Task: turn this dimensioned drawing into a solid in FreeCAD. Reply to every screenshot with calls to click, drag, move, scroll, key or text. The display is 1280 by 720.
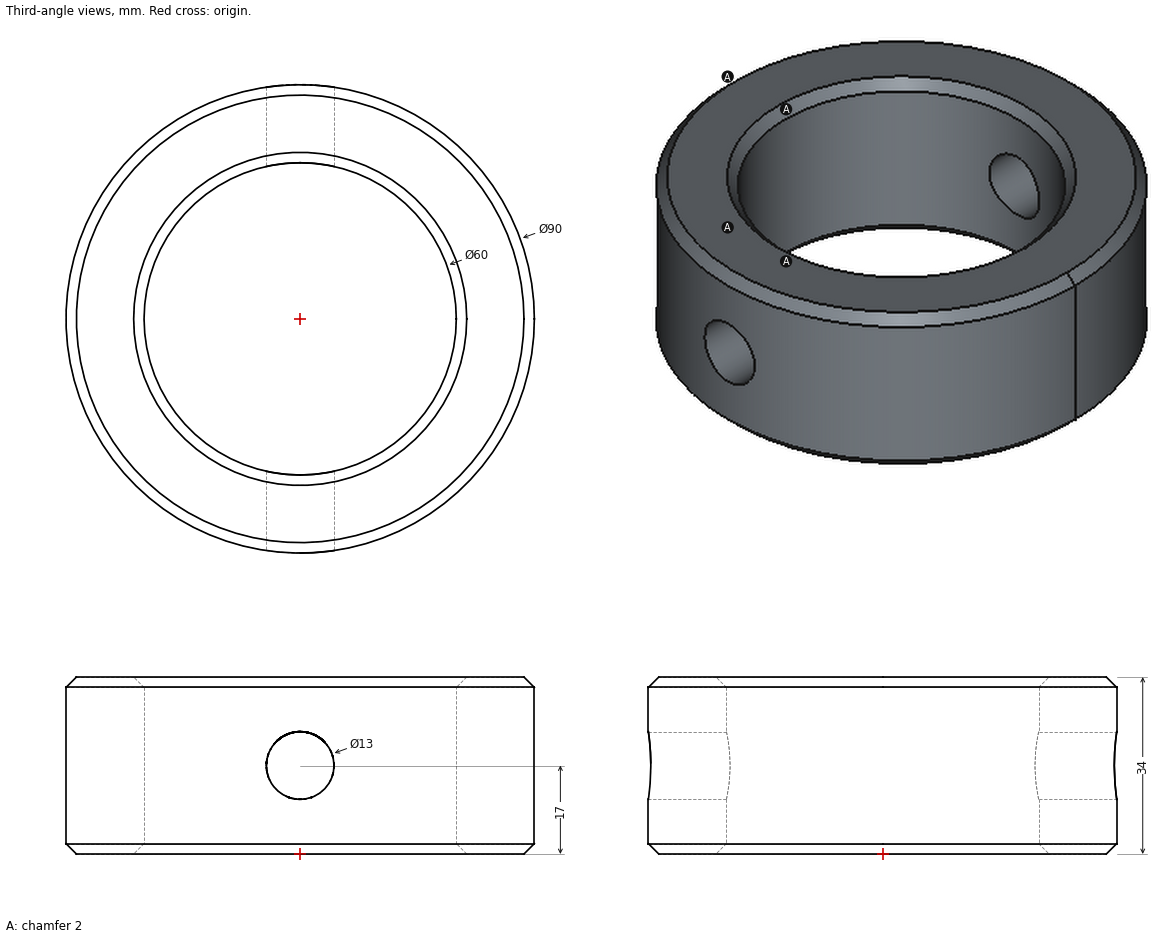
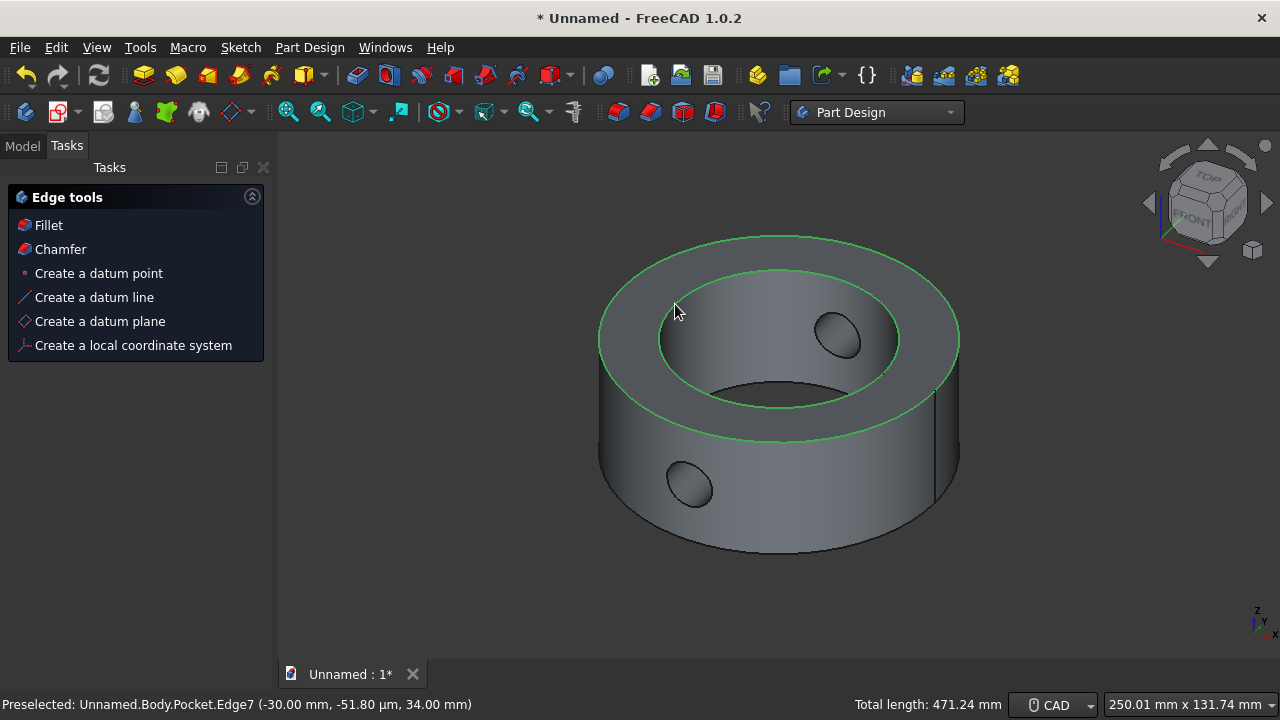
key(0)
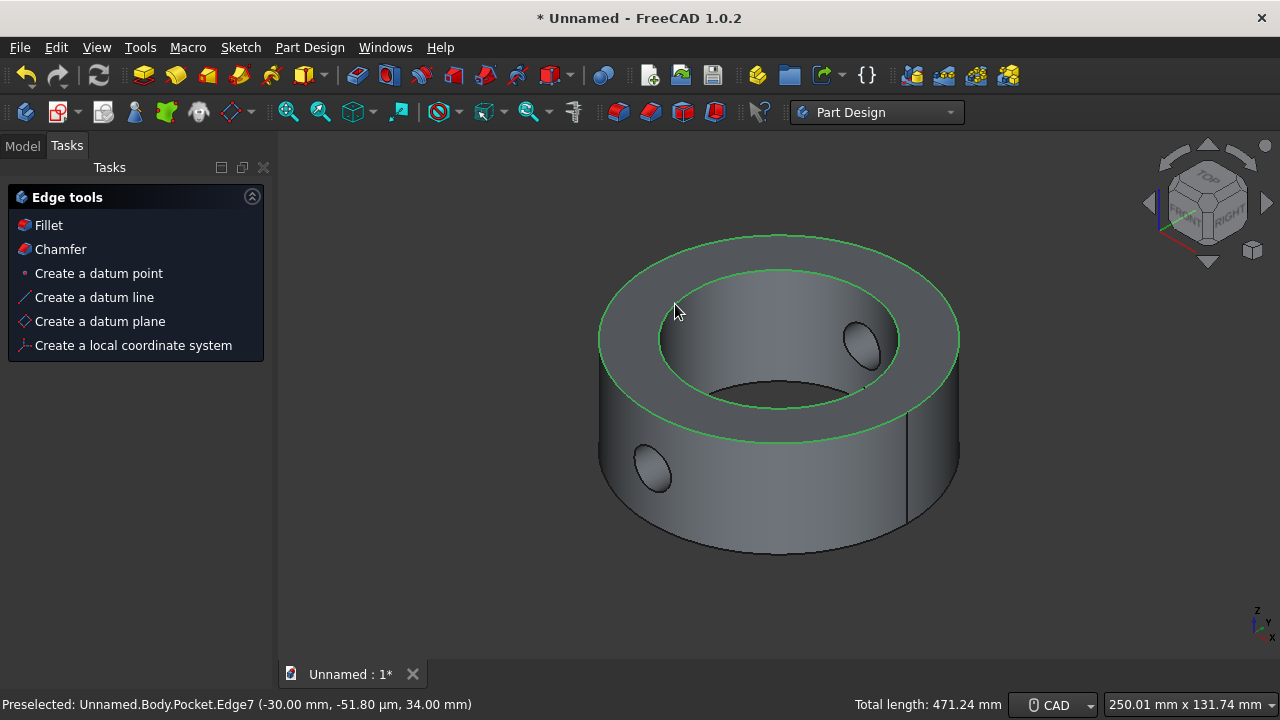
key(2)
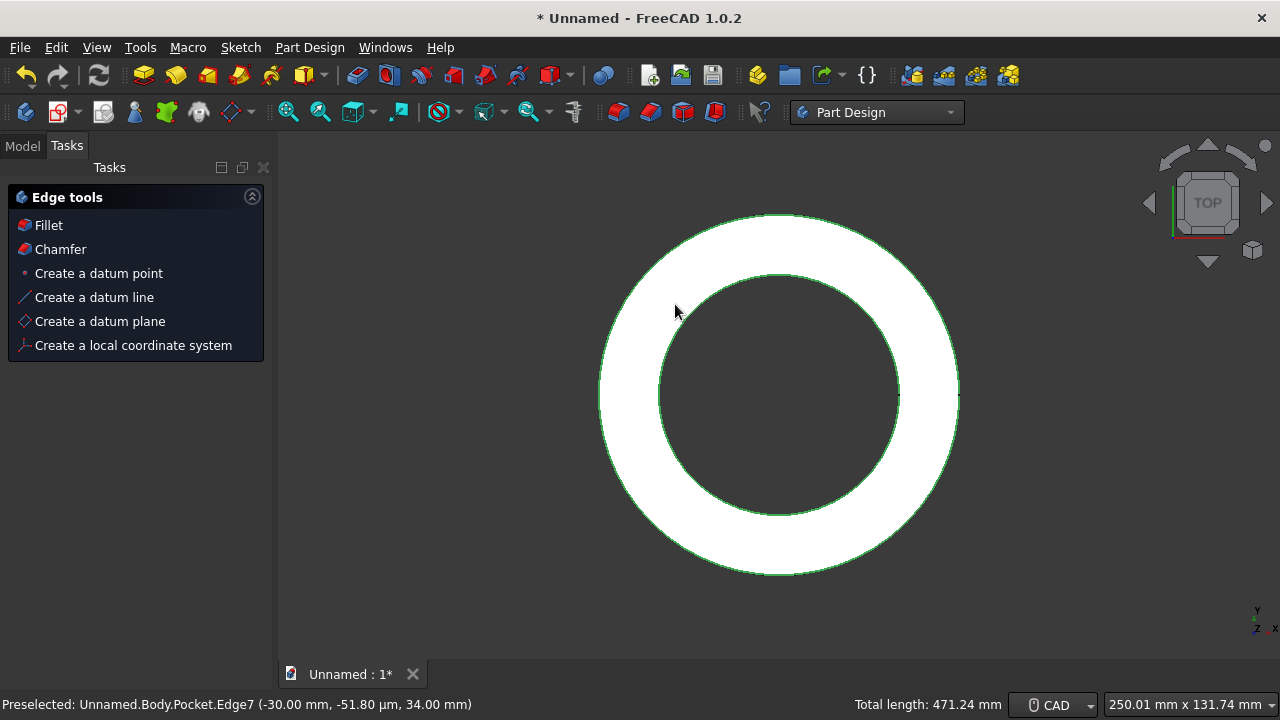
key(1)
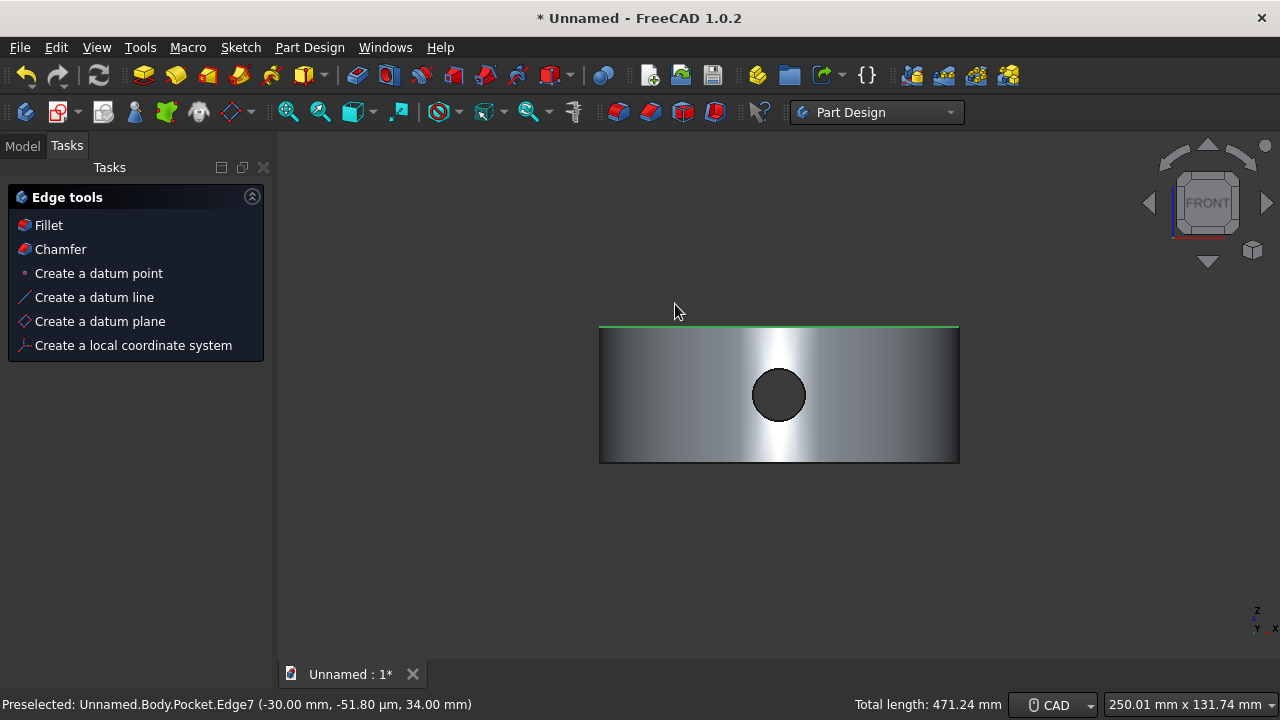
click(290, 112)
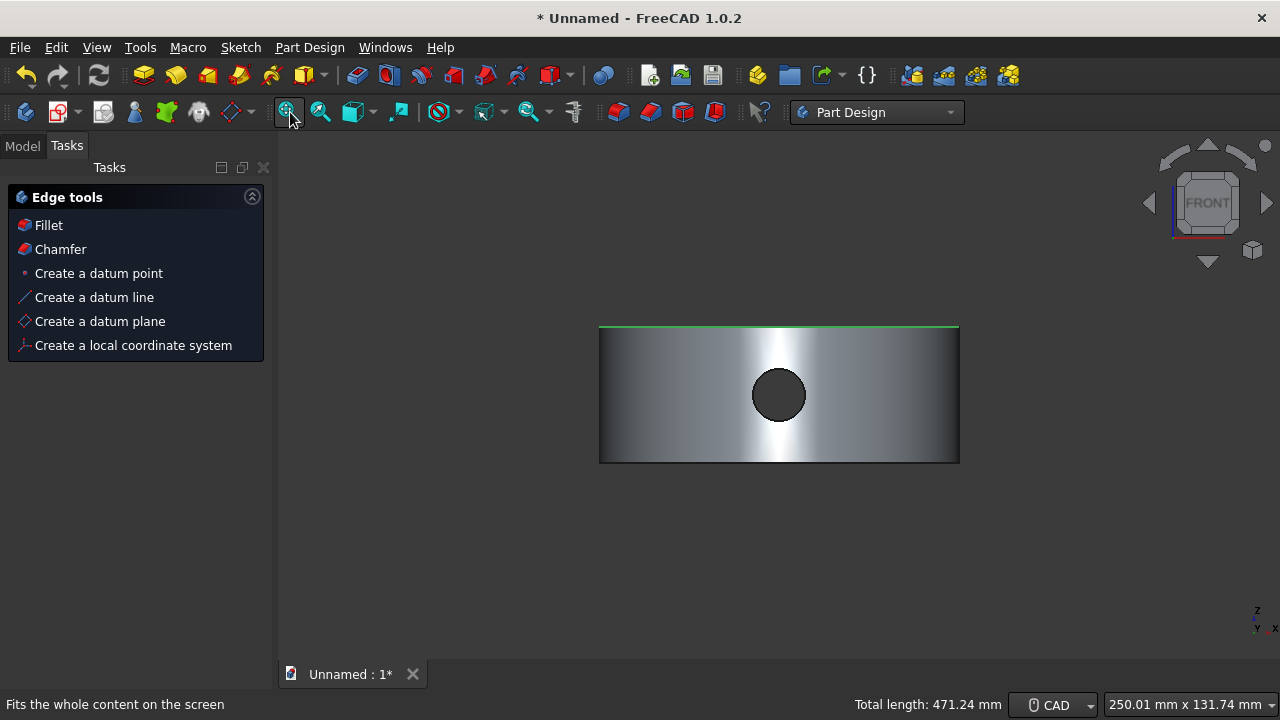
click(633, 462, ctrl)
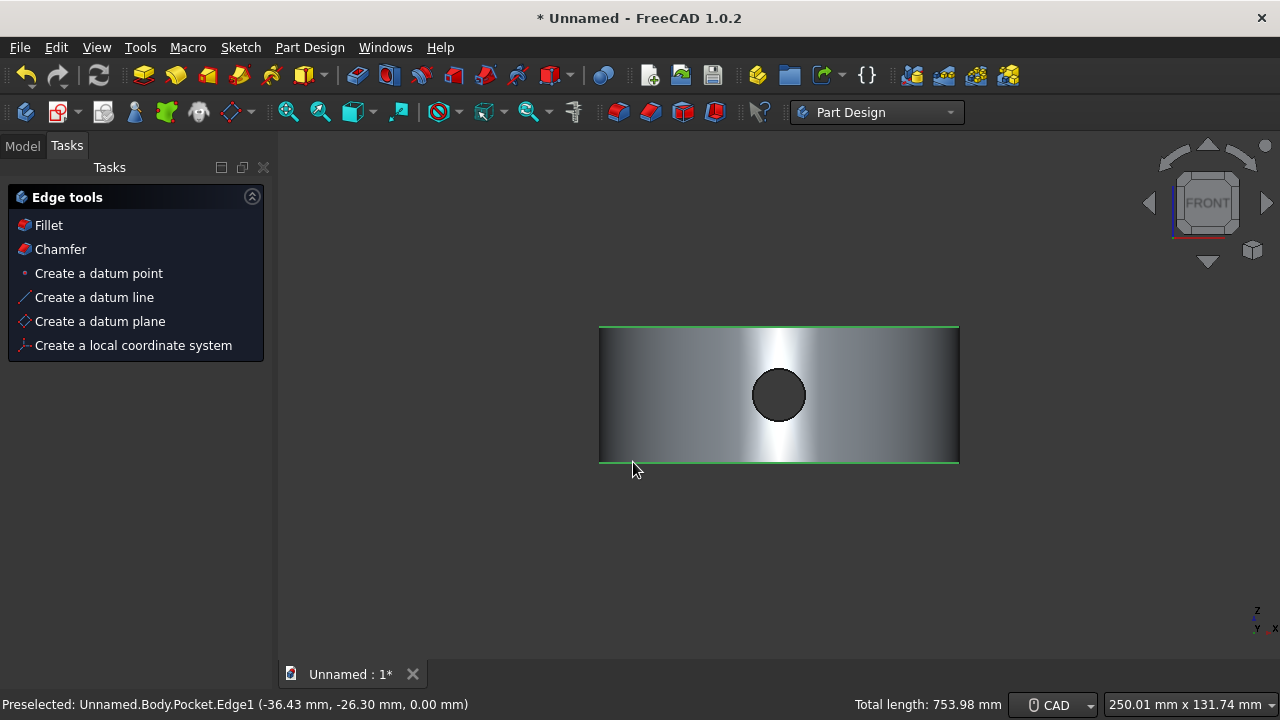
key(3)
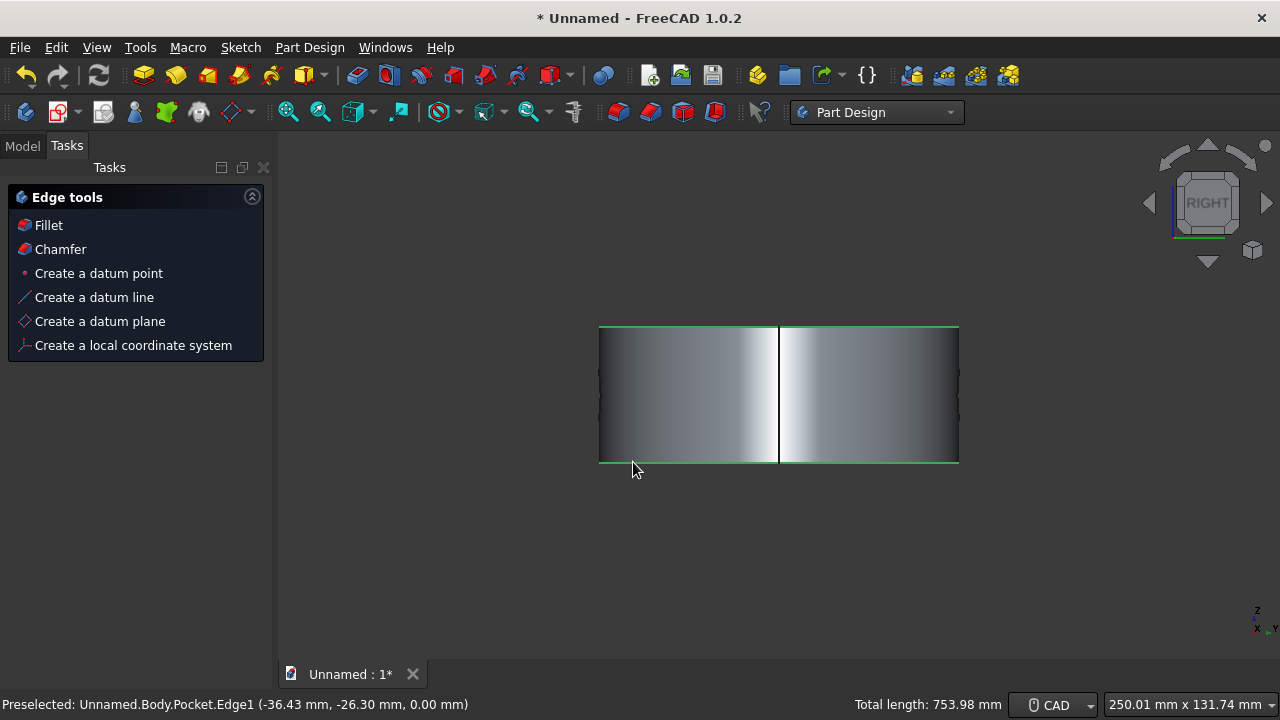
click(290, 112)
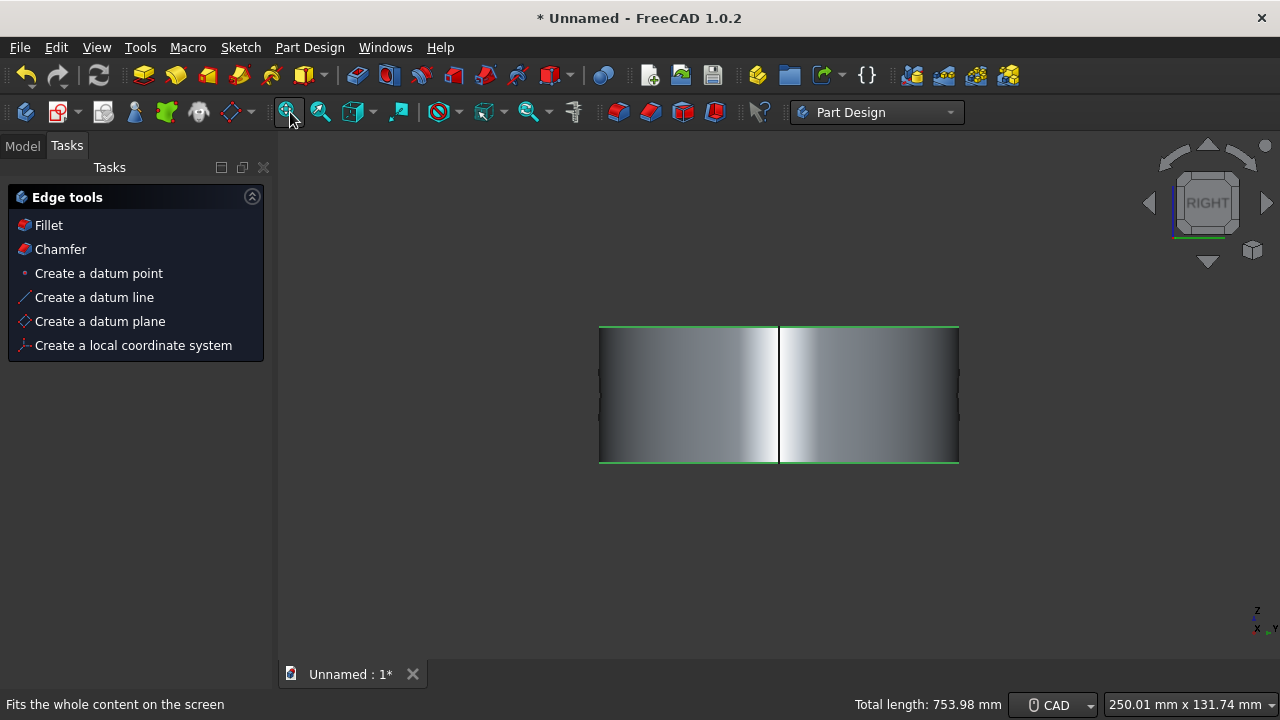
key(5)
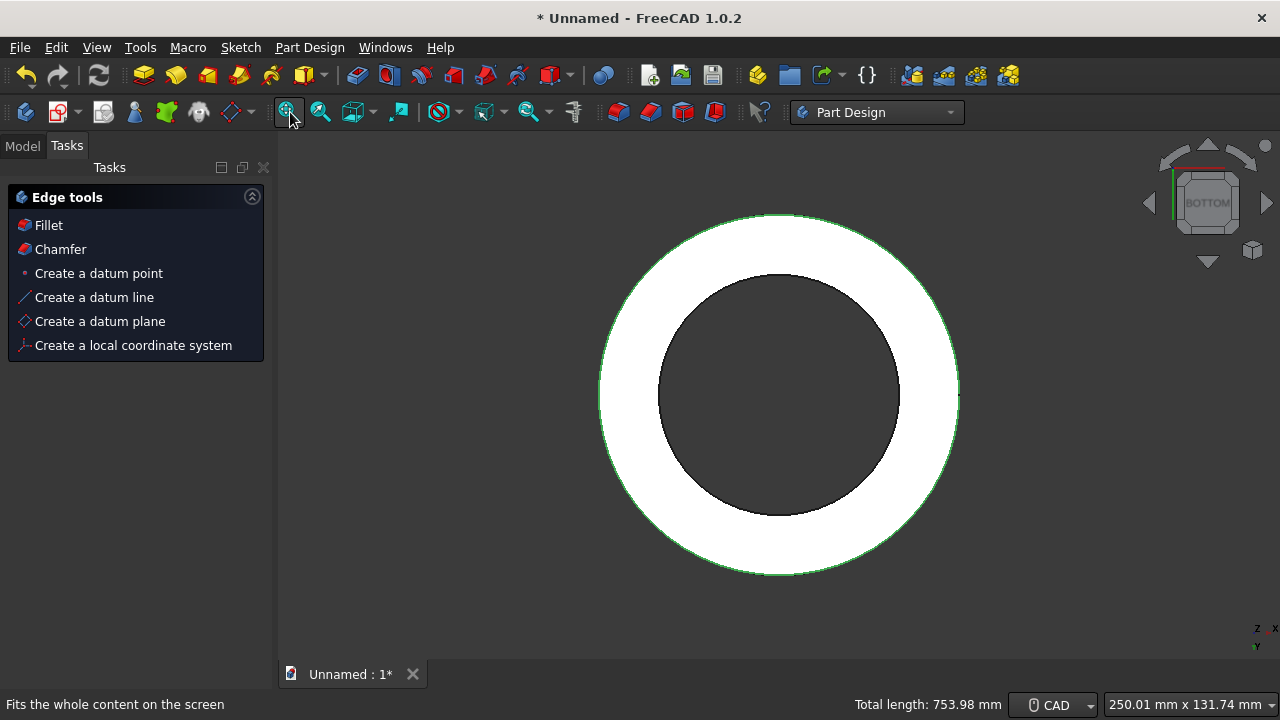
click(682, 465, ctrl)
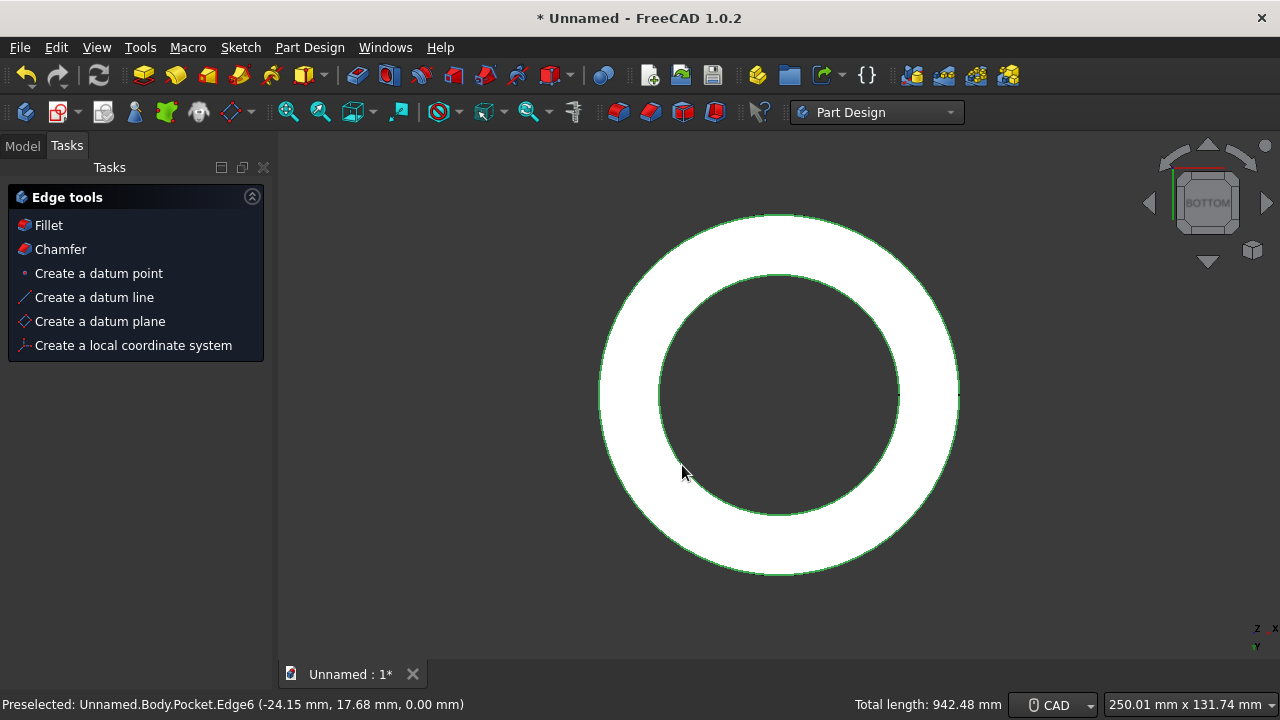
click(652, 112)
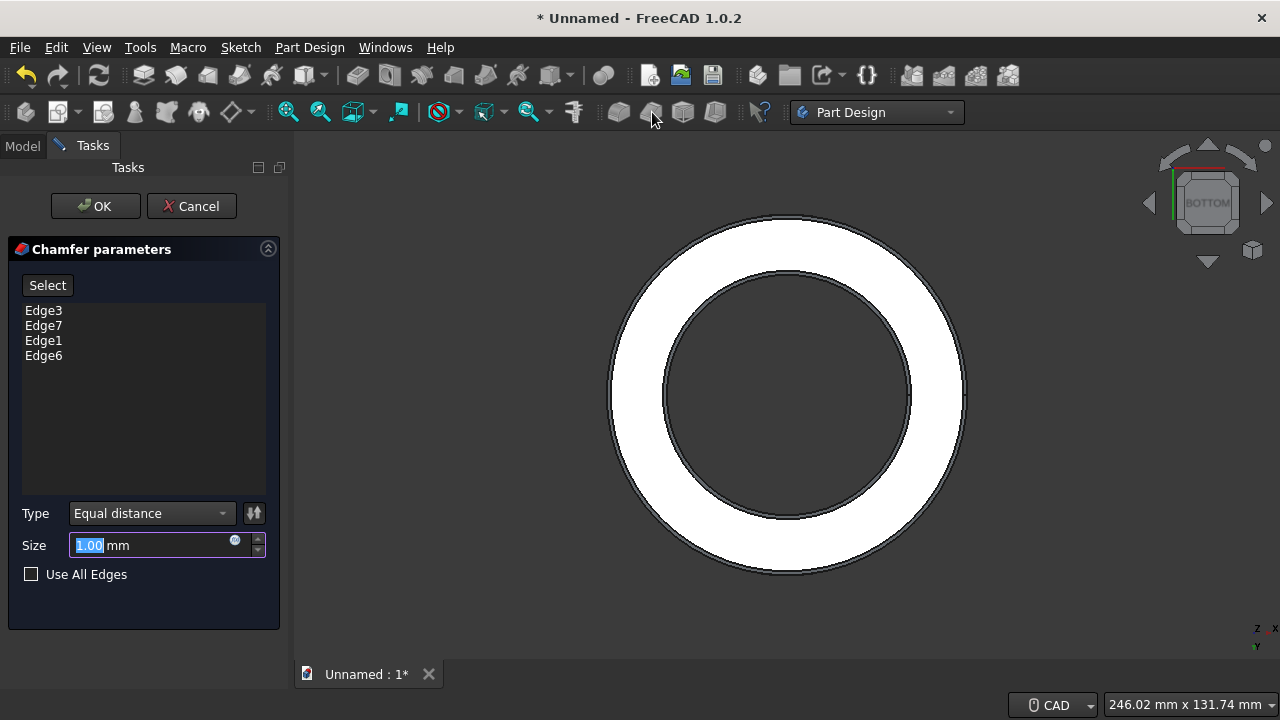
text(2)
key(Tab)